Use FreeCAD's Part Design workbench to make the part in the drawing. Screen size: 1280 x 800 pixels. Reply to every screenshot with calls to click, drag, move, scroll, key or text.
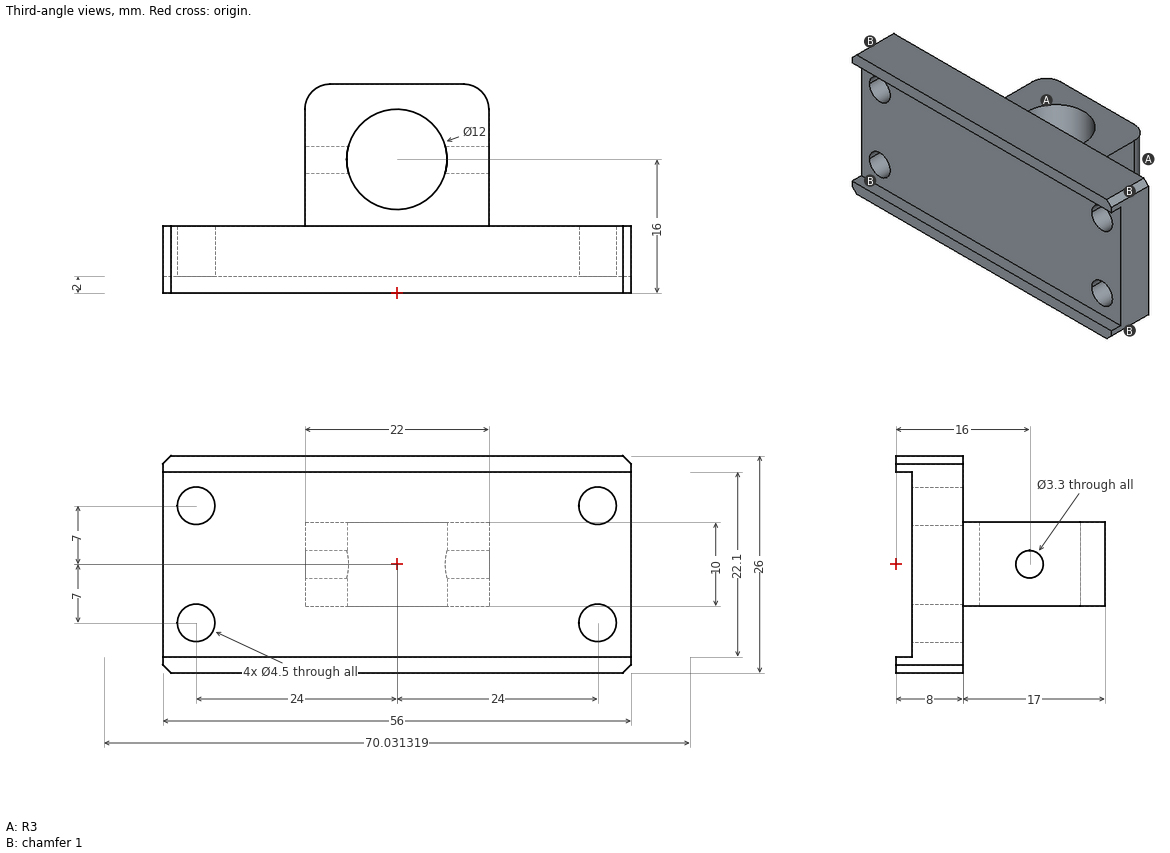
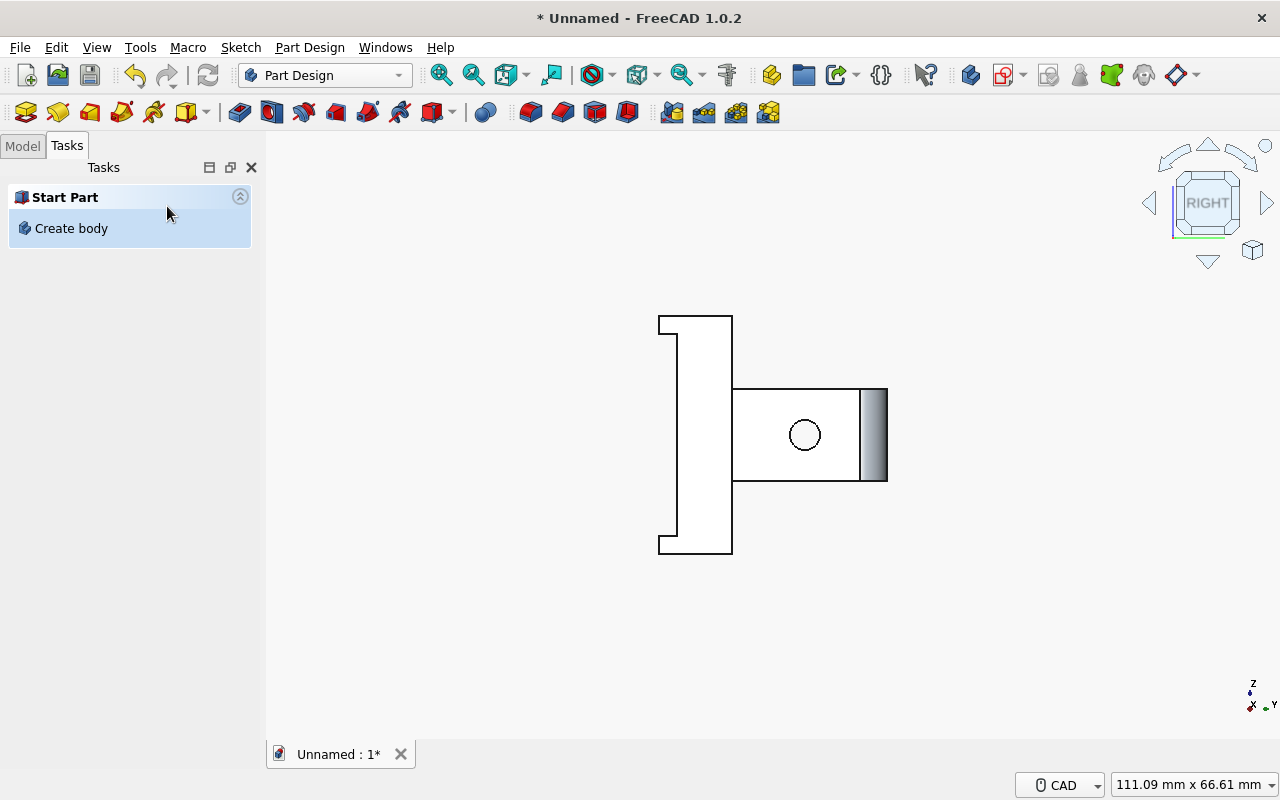
click(442, 76)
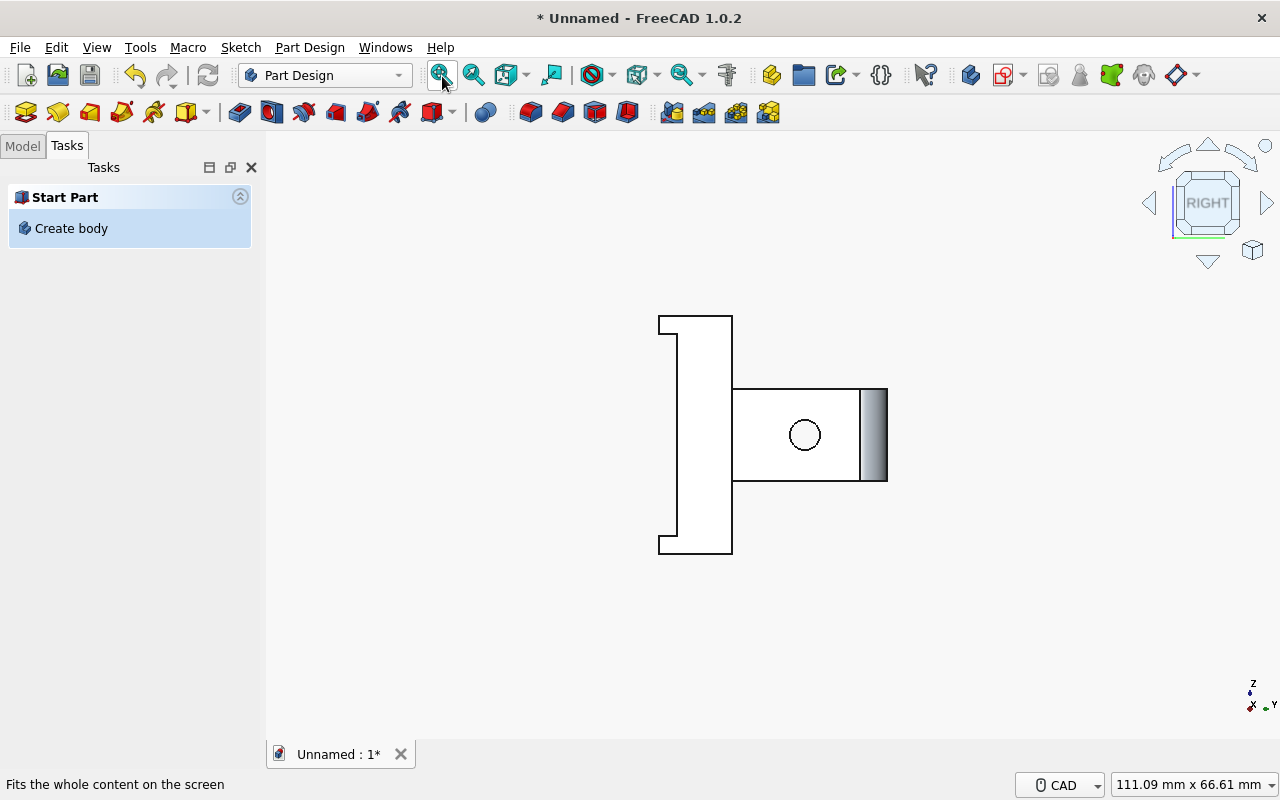
click(695, 553)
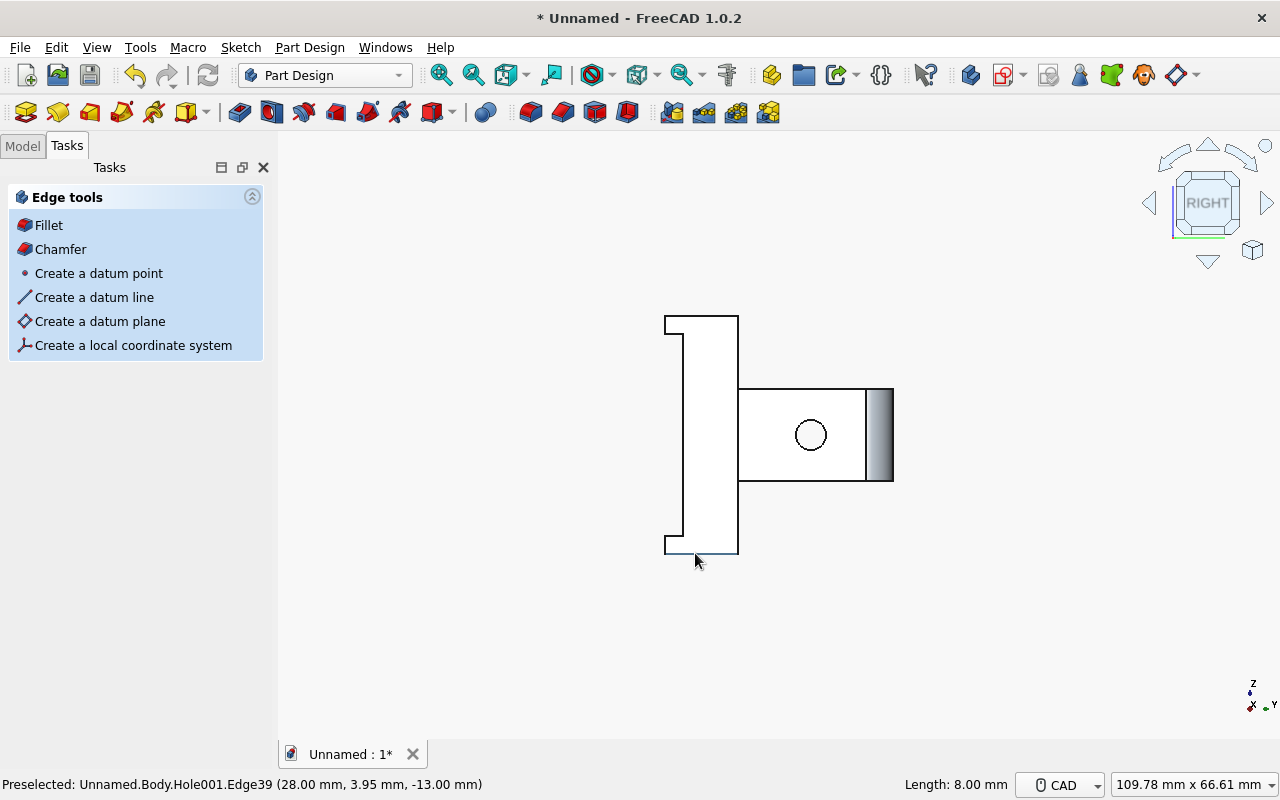
key(0)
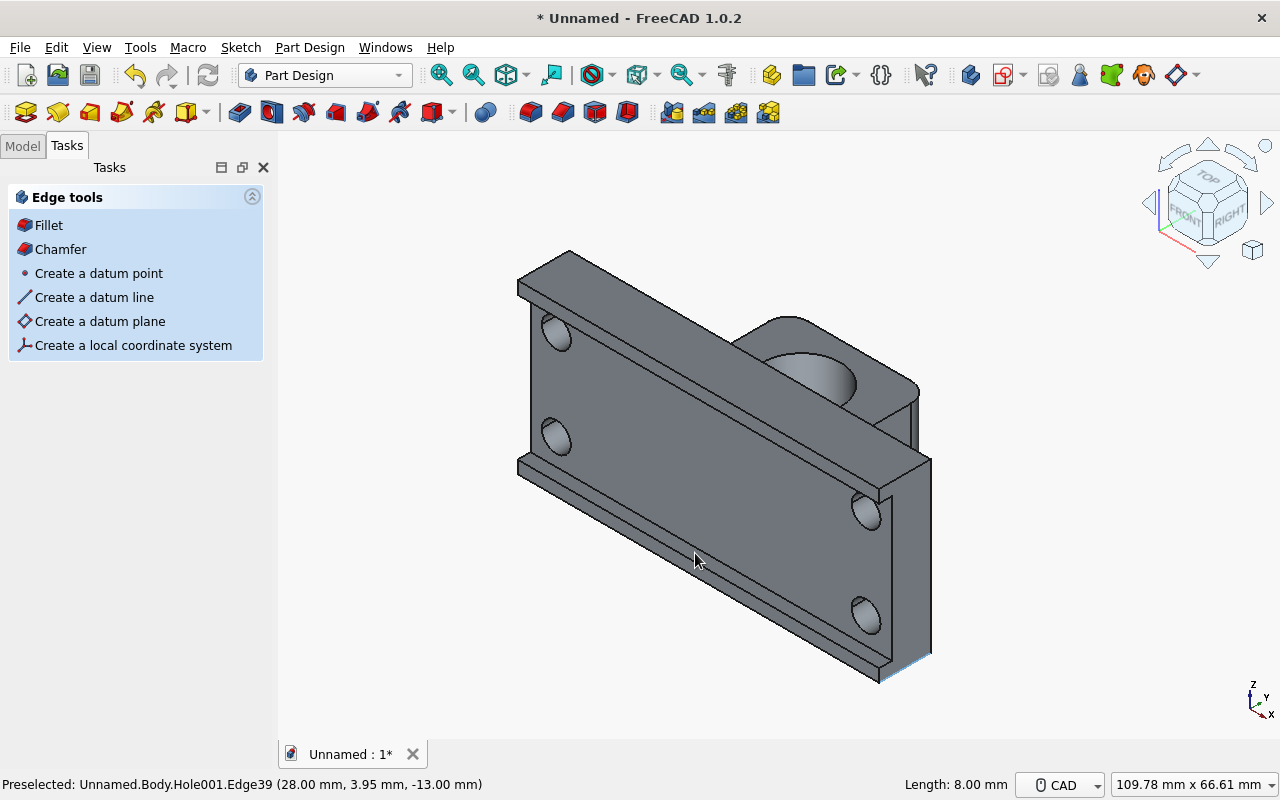
click(905, 473, ctrl)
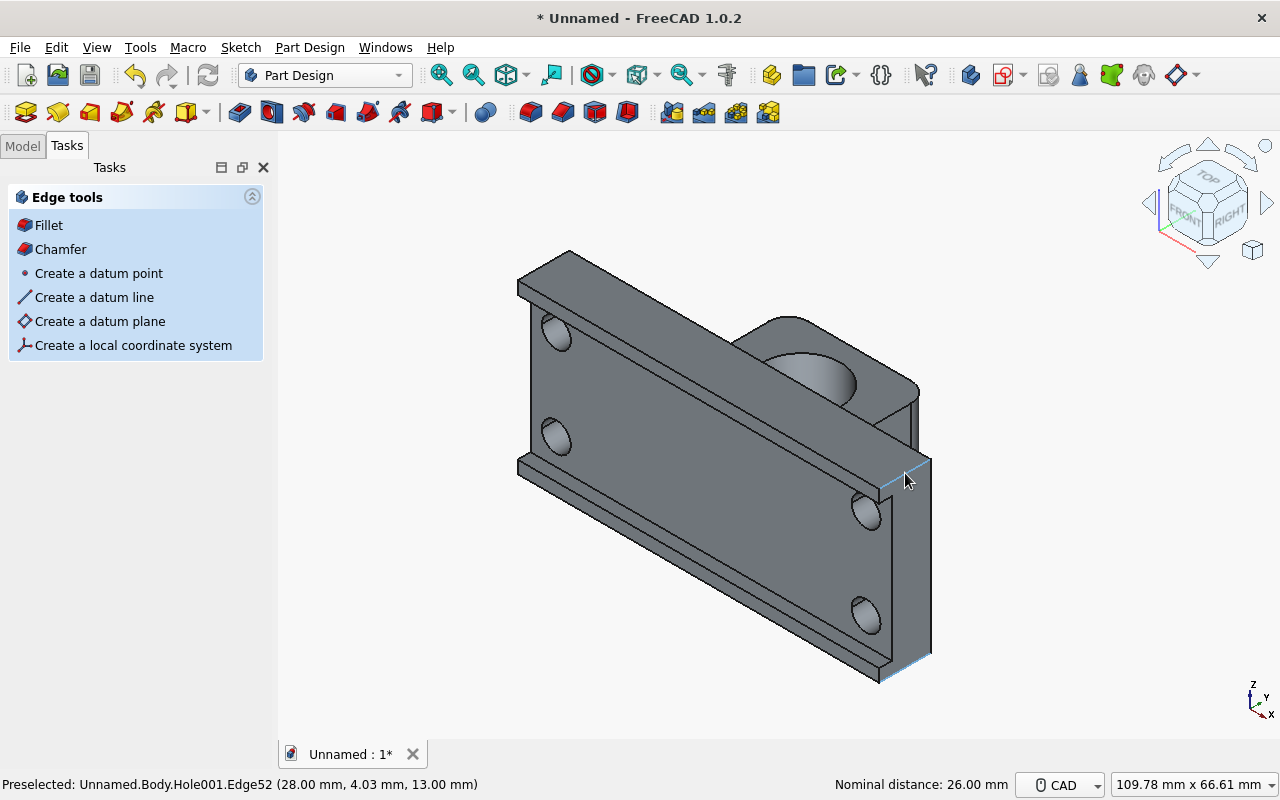
key(2)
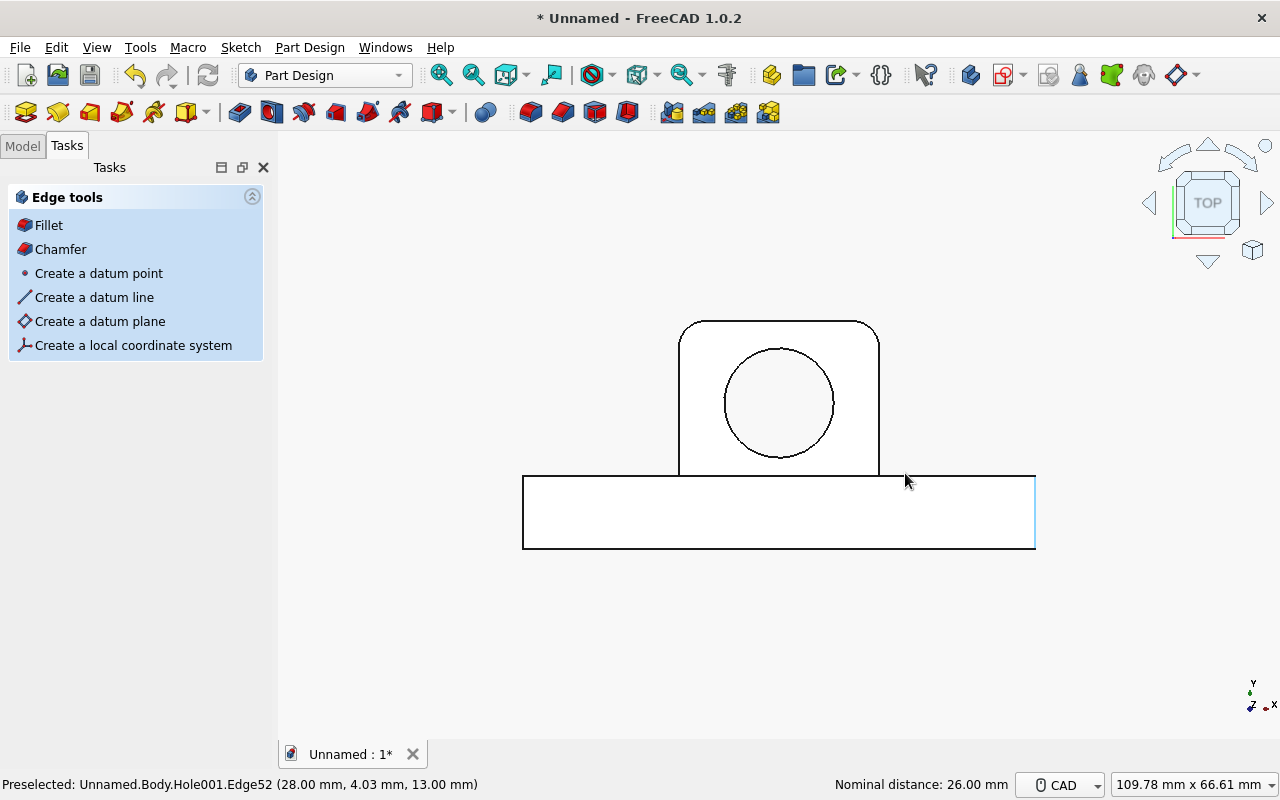
click(523, 512, ctrl)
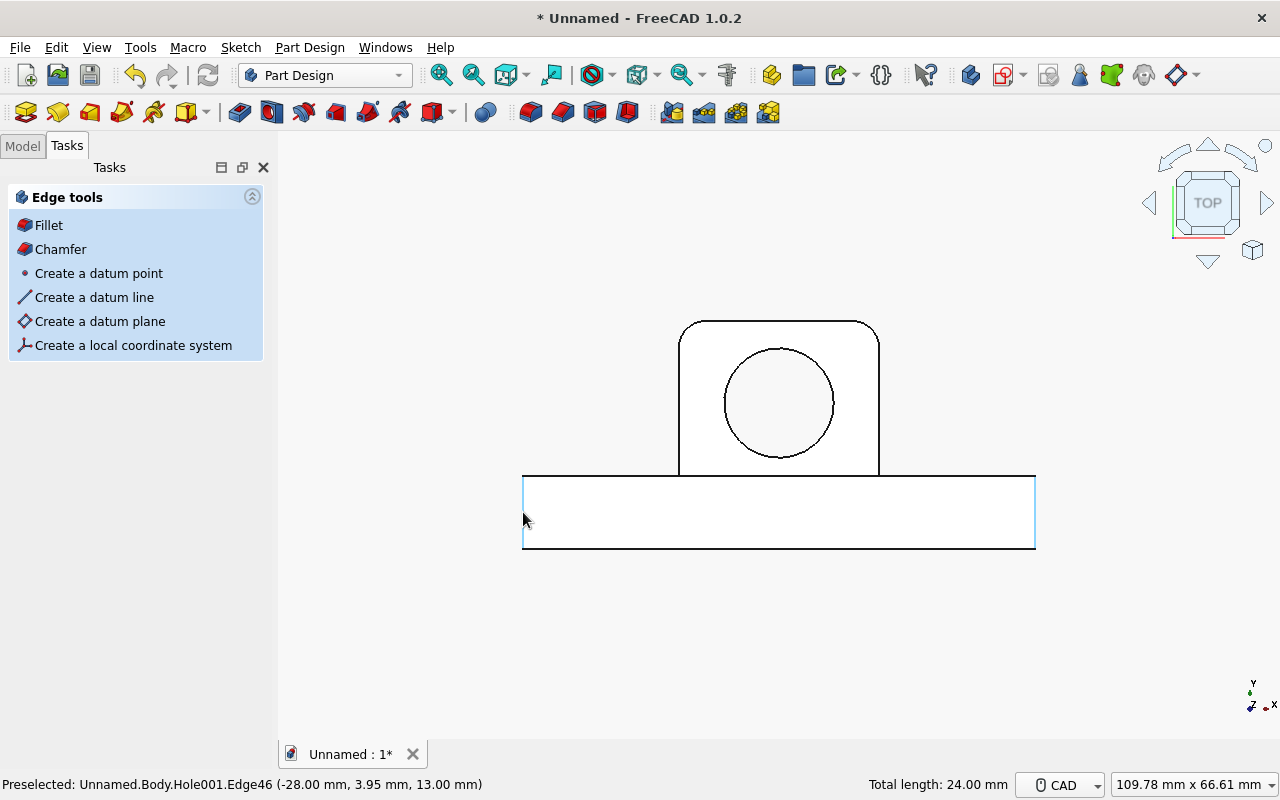
key(1)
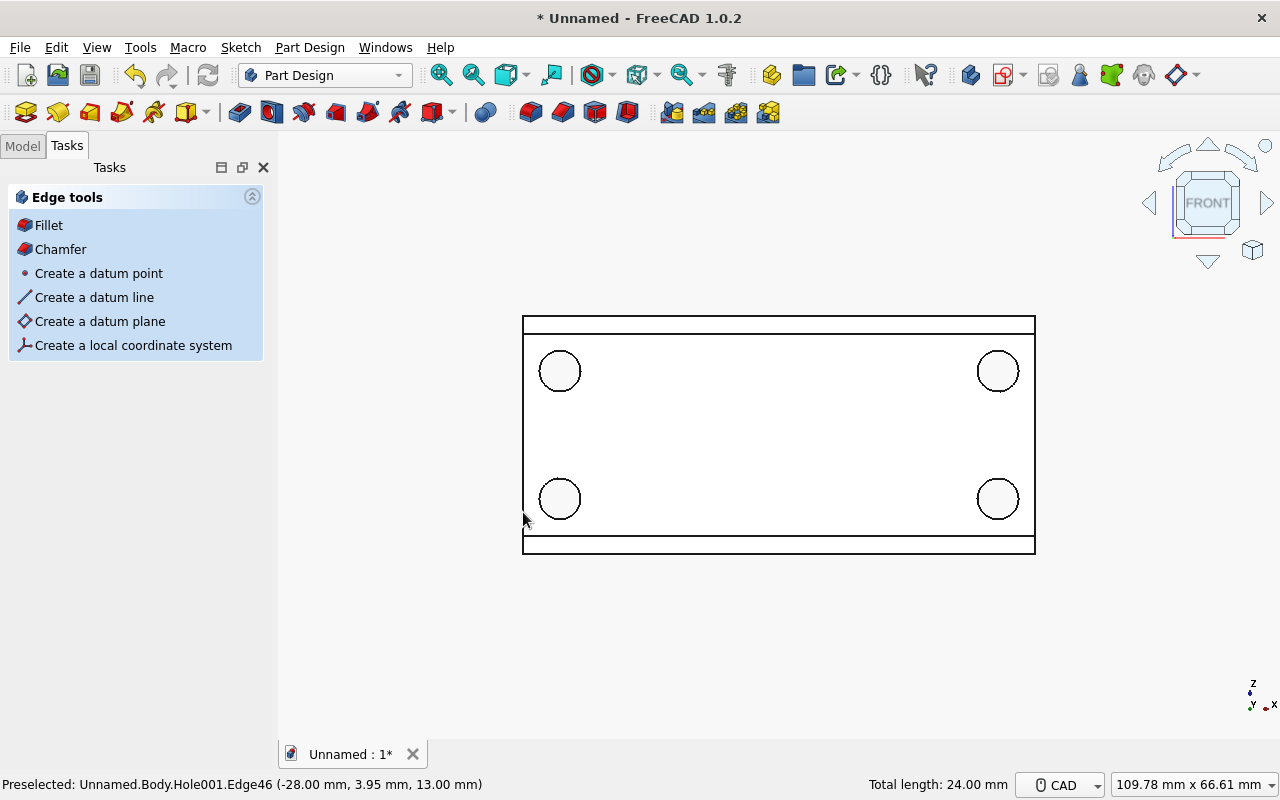
key(3)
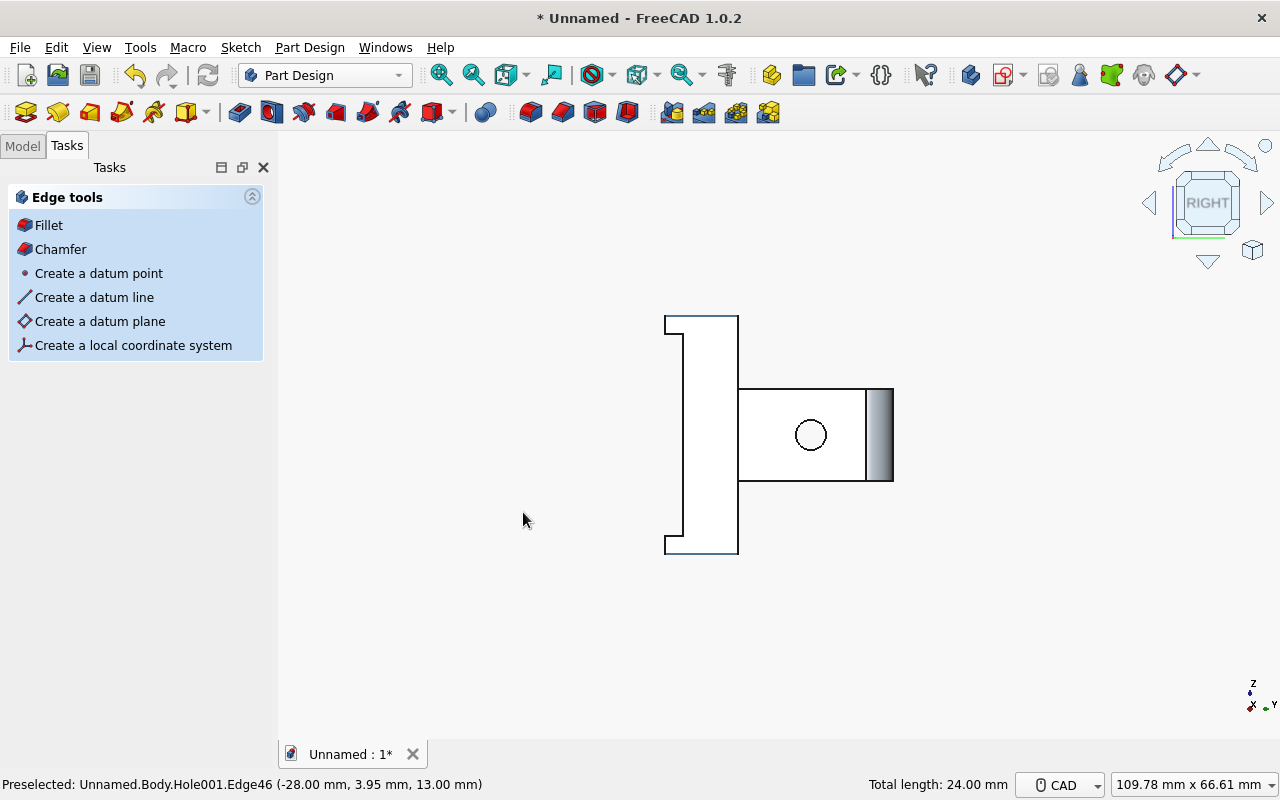
click(442, 76)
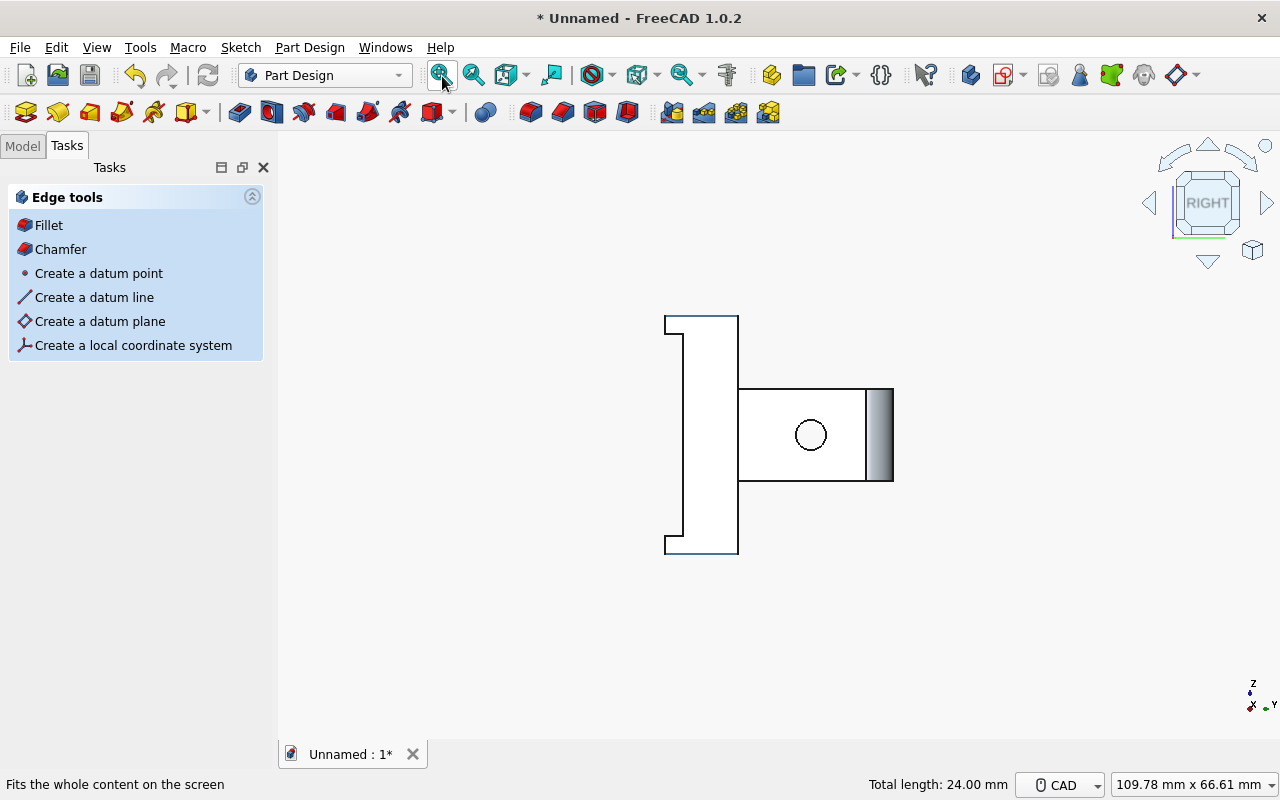
key(5)